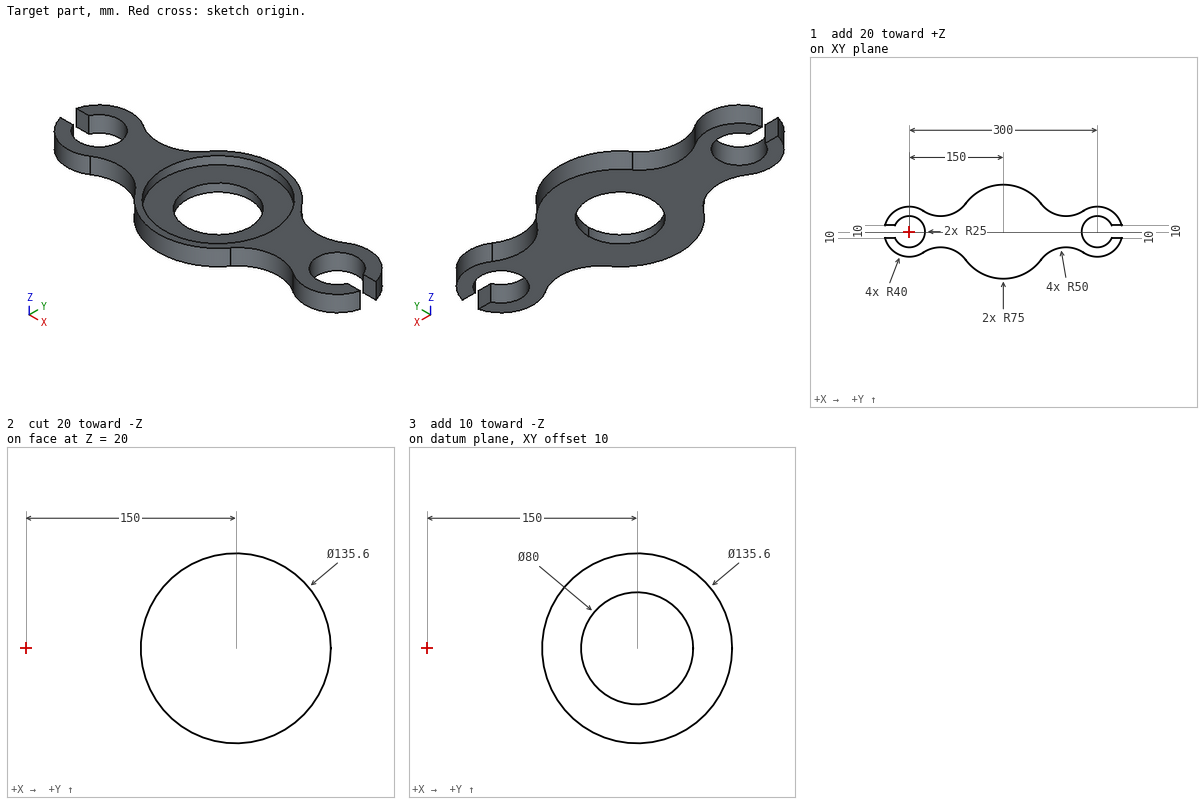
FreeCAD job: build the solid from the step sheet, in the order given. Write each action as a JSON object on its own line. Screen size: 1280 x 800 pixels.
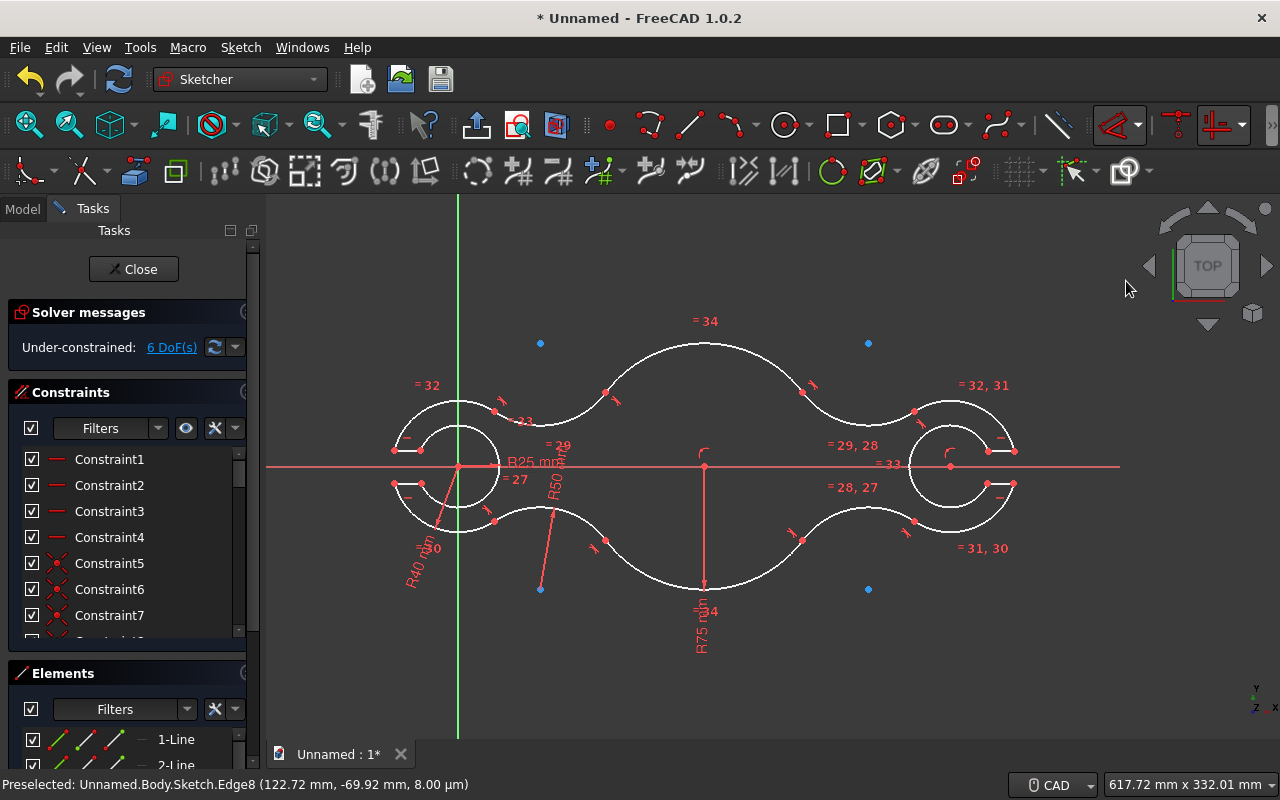
{"action": "scroll", "coordinate": [394, 451], "scroll_direction": "up", "scroll_amount": 5}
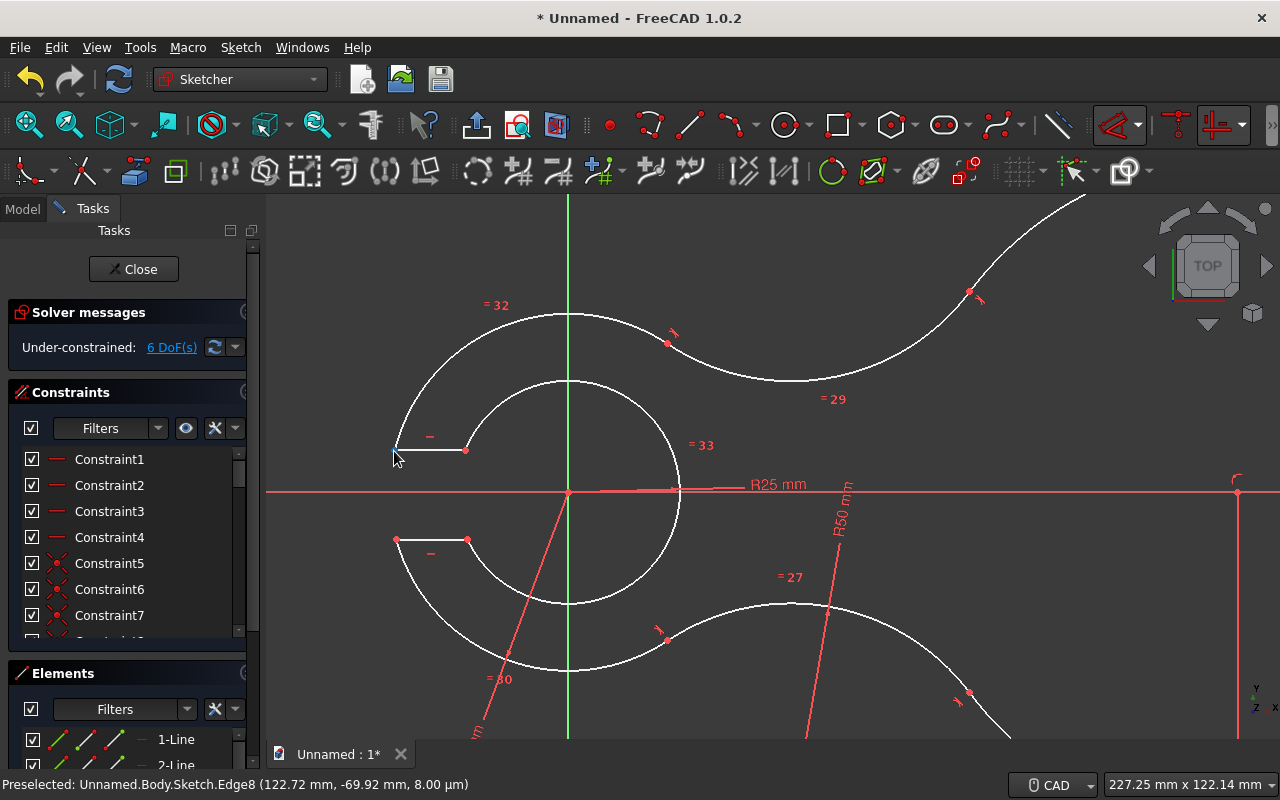
{"action": "left_click", "coordinate": [395, 450]}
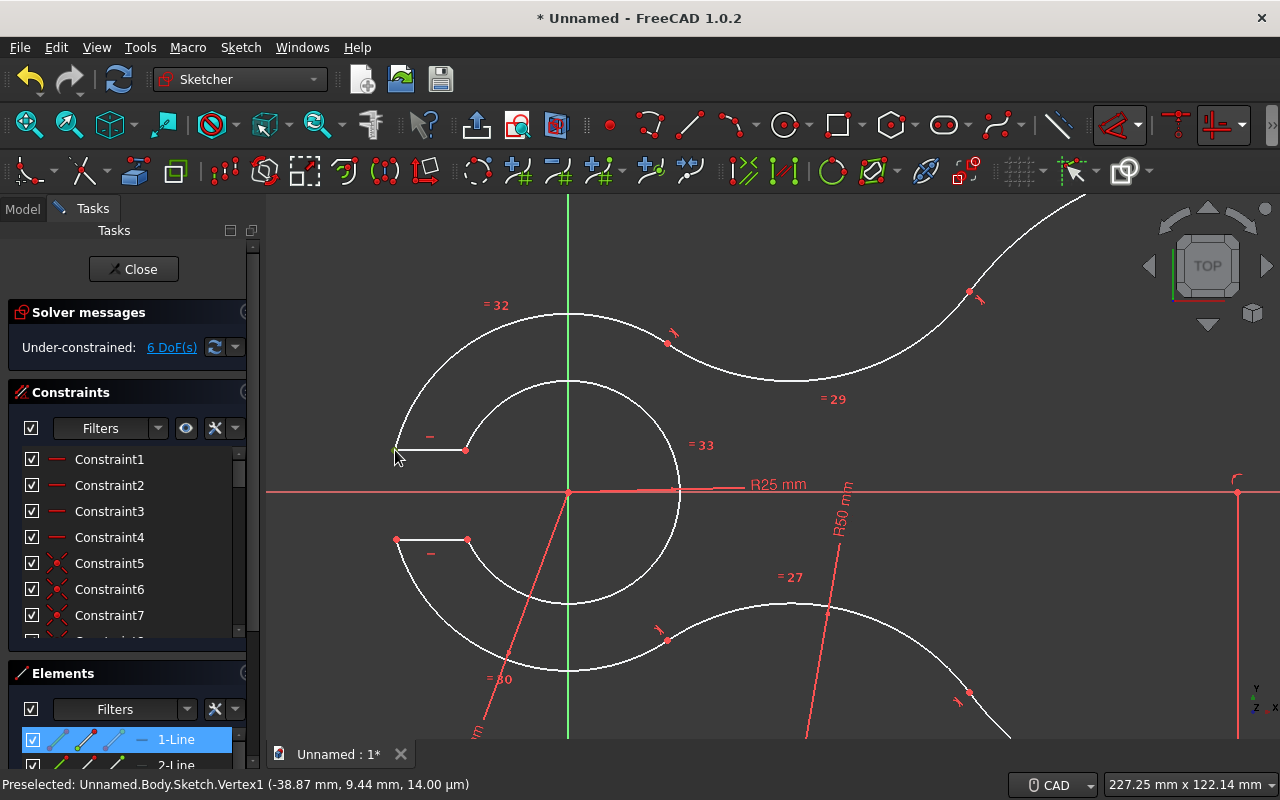
{"action": "left_click", "coordinate": [1140, 126]}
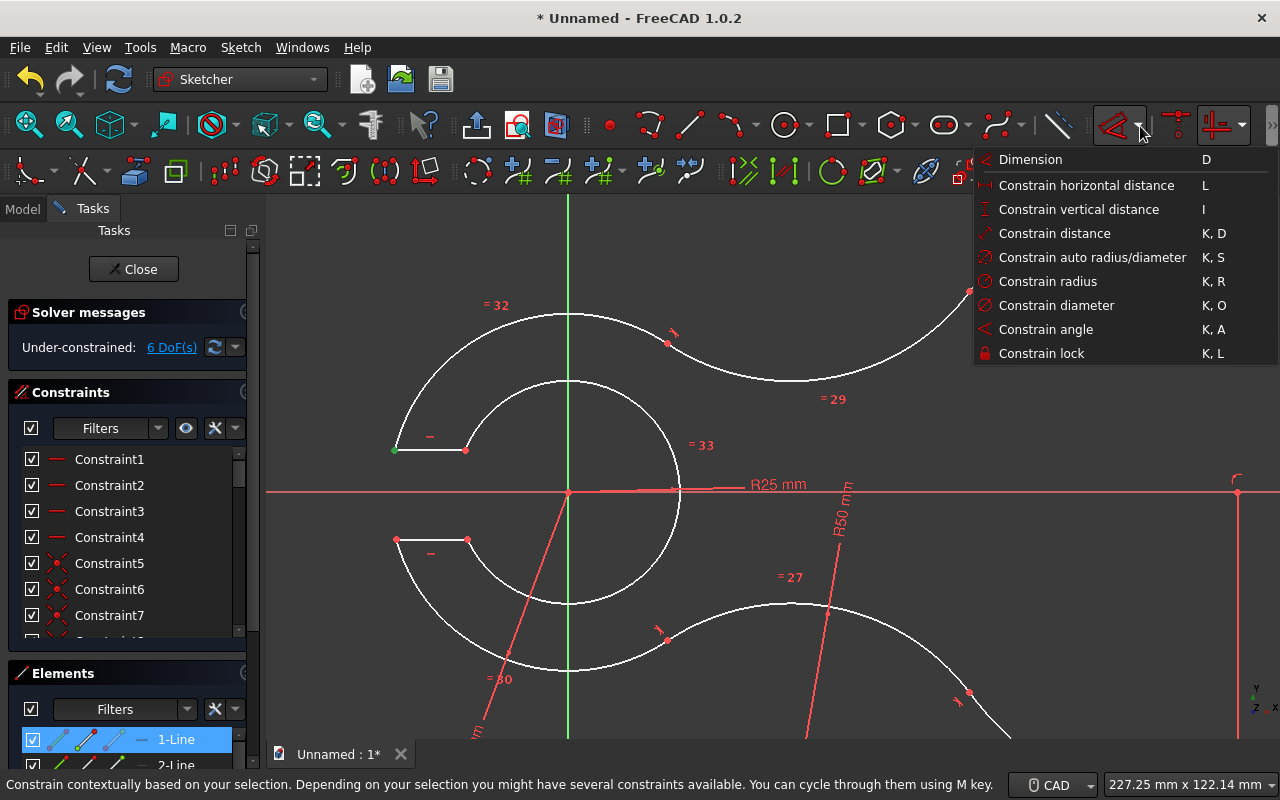
{"action": "left_click", "coordinate": [1126, 209]}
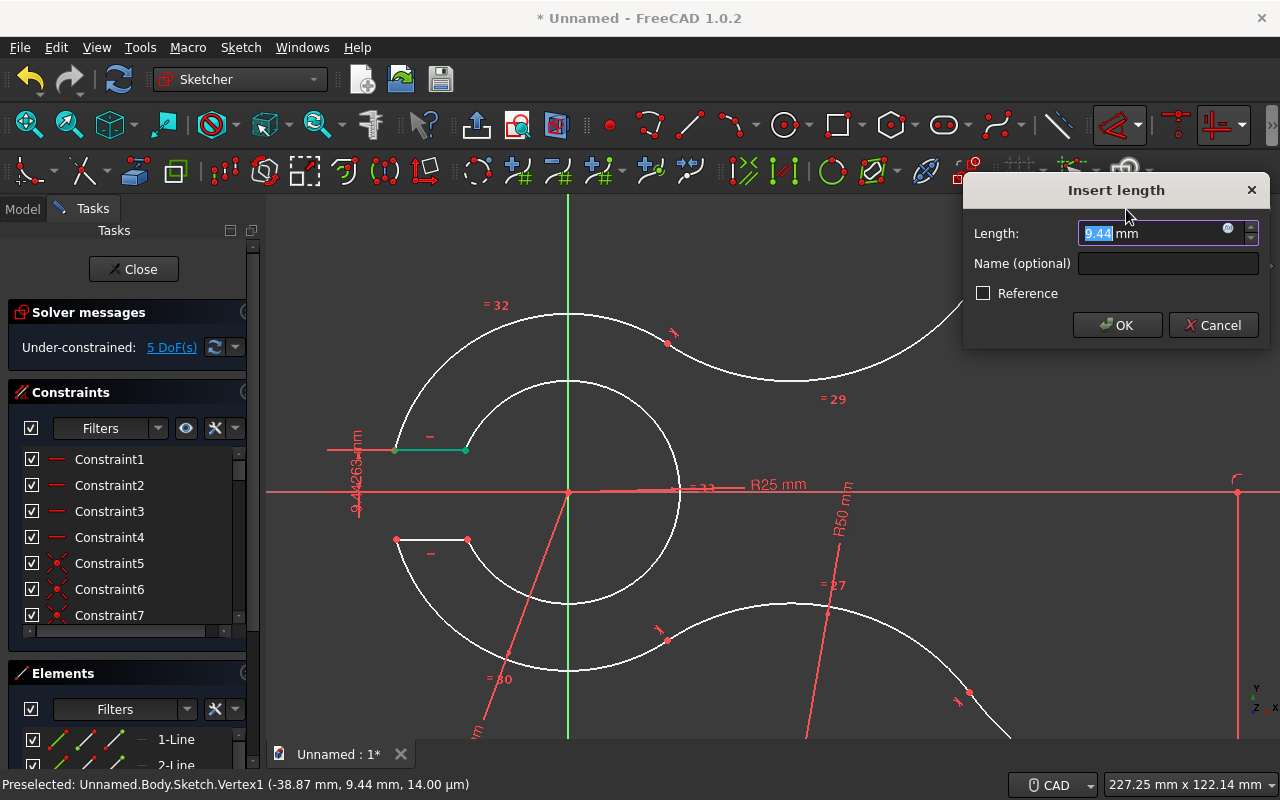
{"action": "type", "text": "10"}
{"action": "key", "text": "Return"}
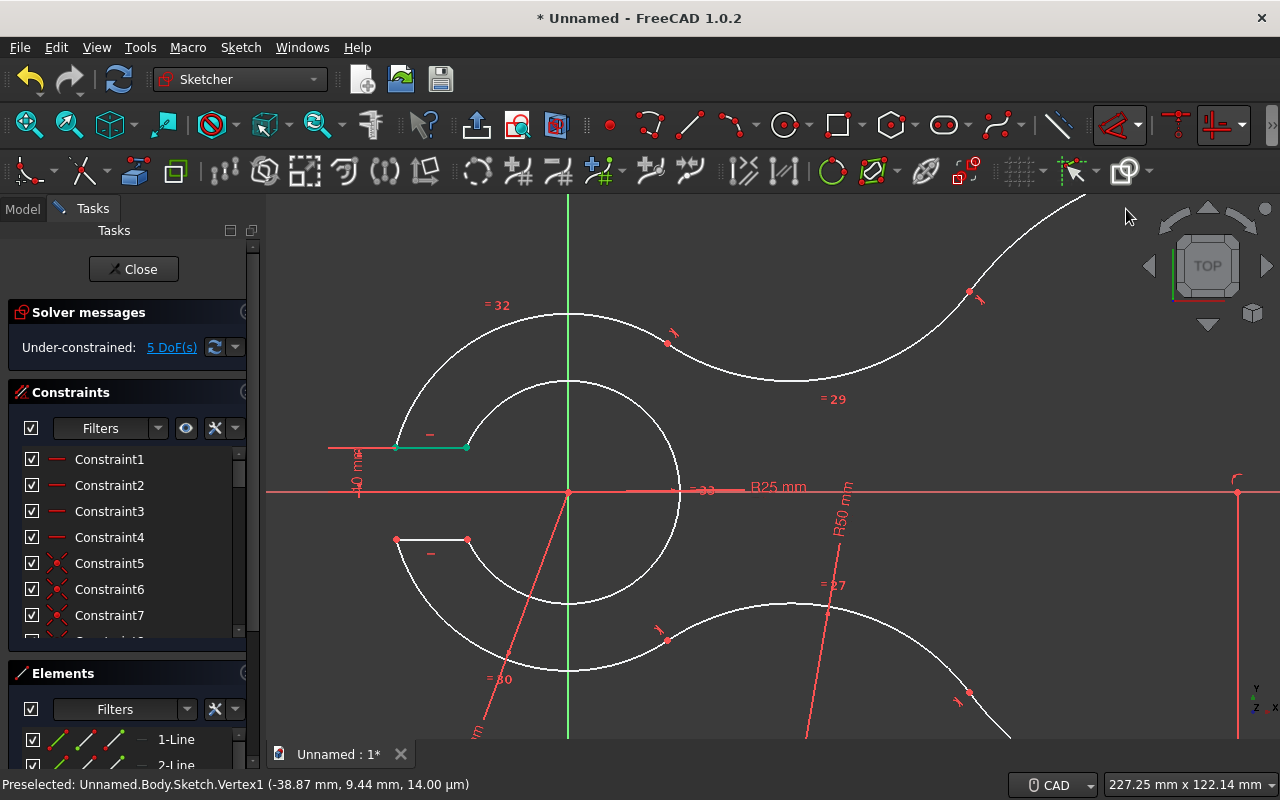
{"action": "left_click", "coordinate": [467, 540]}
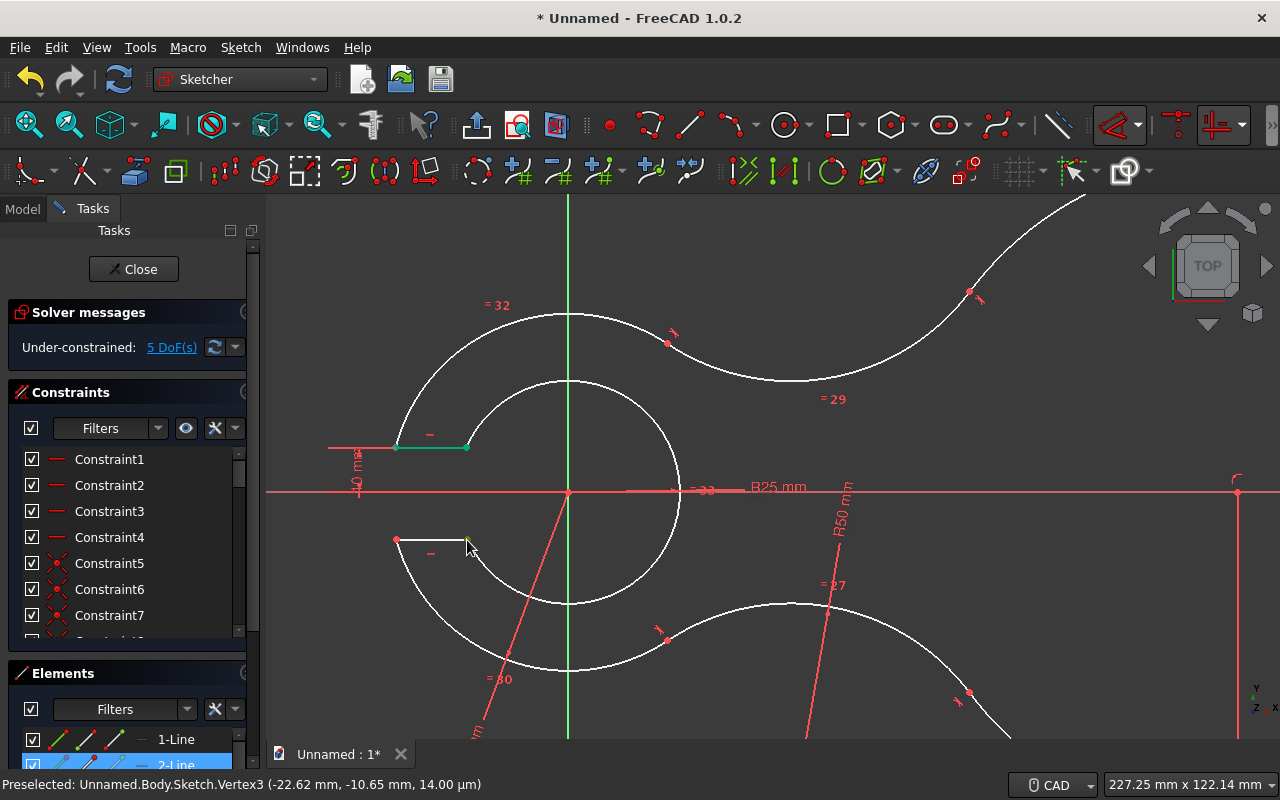
{"action": "key", "text": "i"}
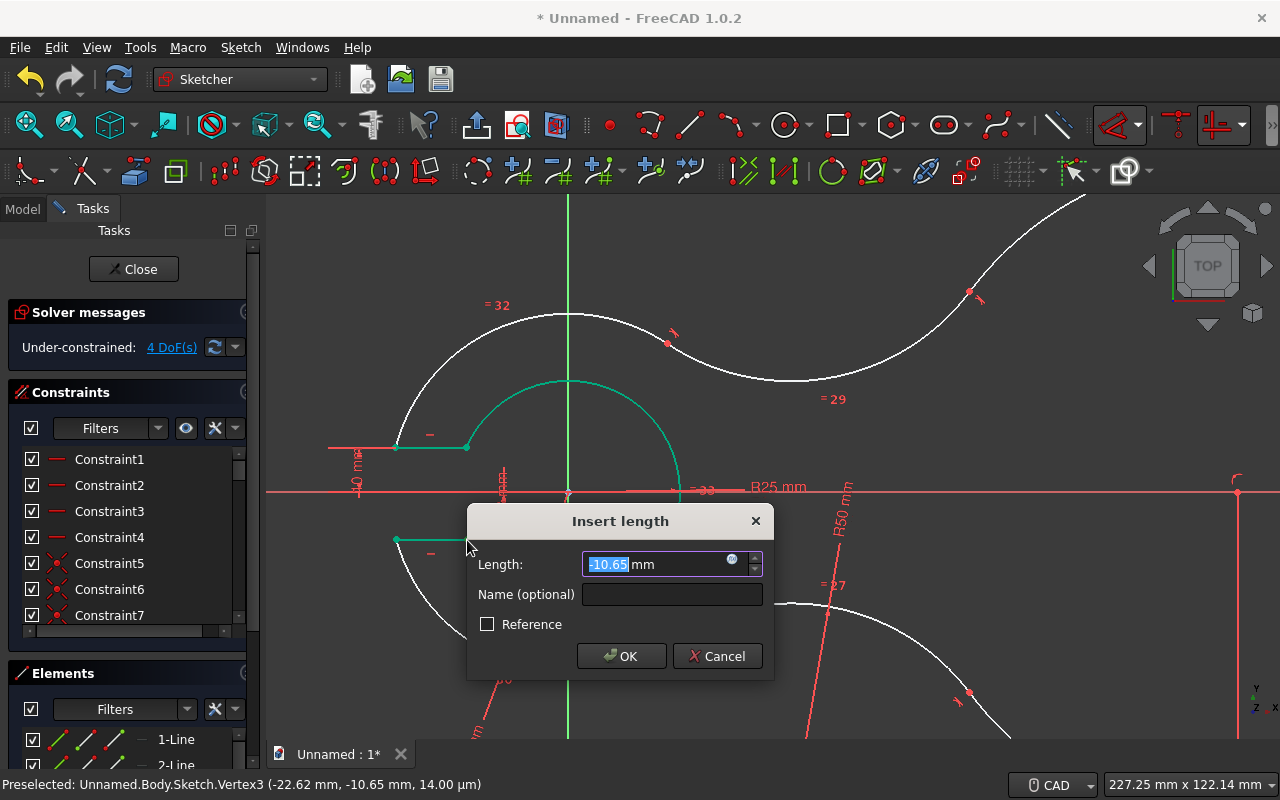
{"action": "type", "text": "-10"}
{"action": "key", "text": "Return"}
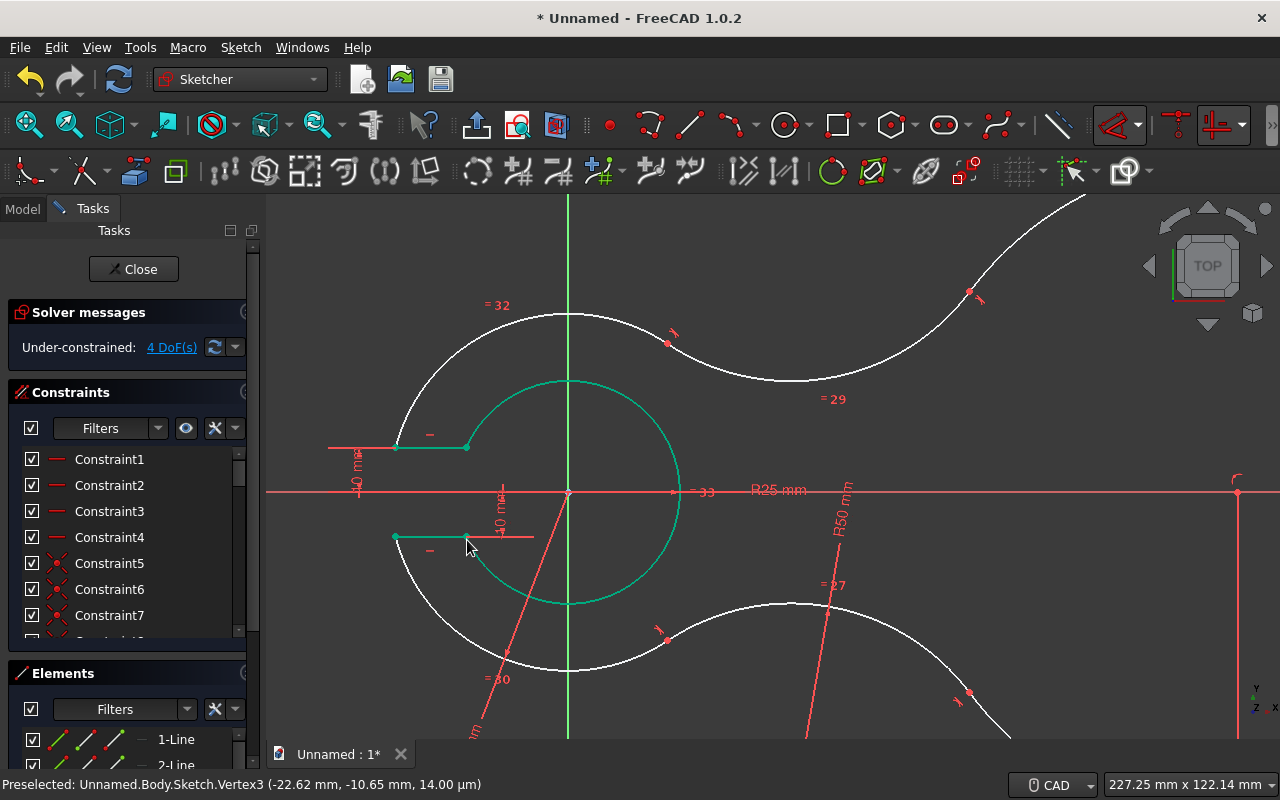
{"action": "scroll", "coordinate": [394, 451], "scroll_direction": "down", "scroll_amount": 5}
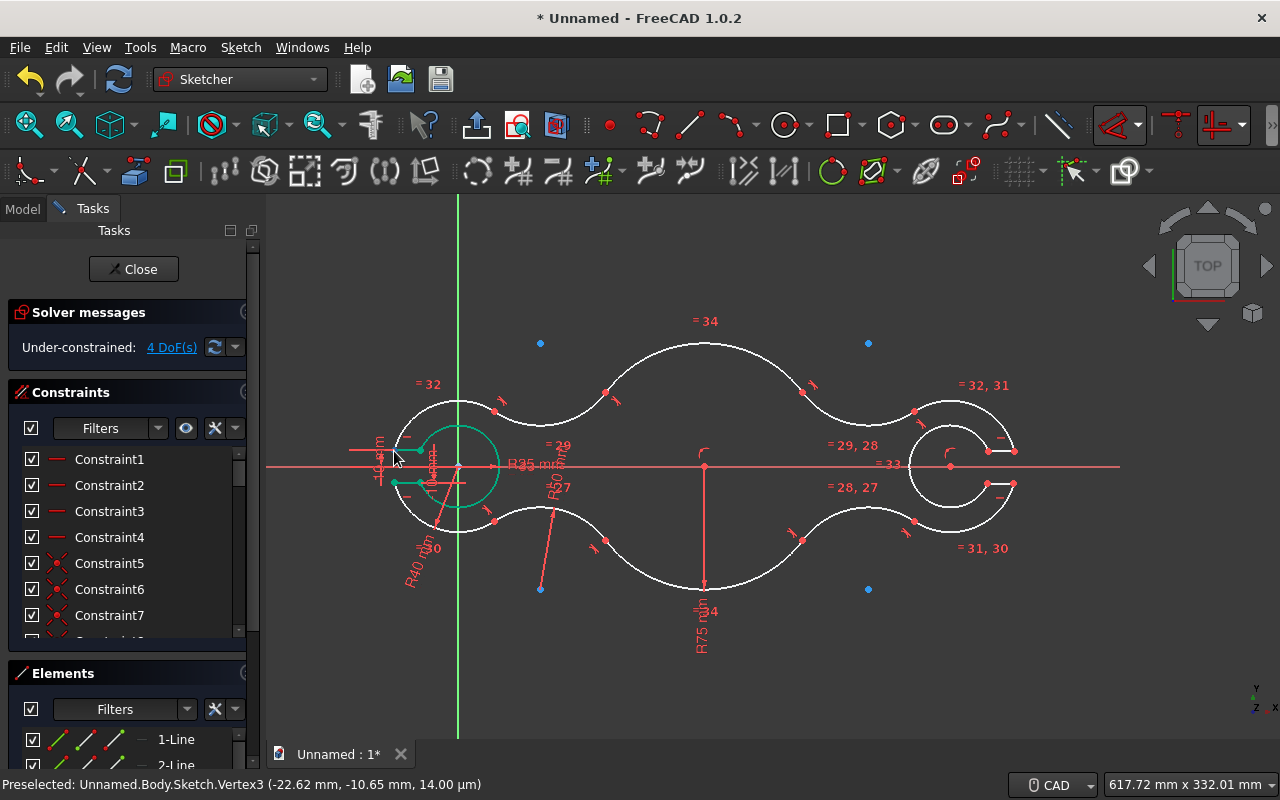
{"action": "scroll", "coordinate": [1014, 484], "scroll_direction": "up", "scroll_amount": 5}